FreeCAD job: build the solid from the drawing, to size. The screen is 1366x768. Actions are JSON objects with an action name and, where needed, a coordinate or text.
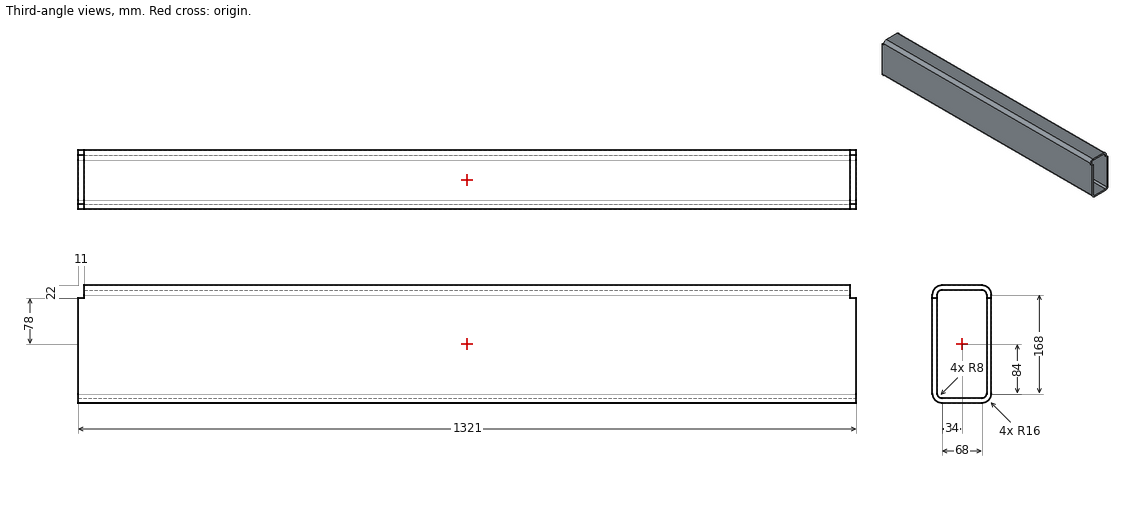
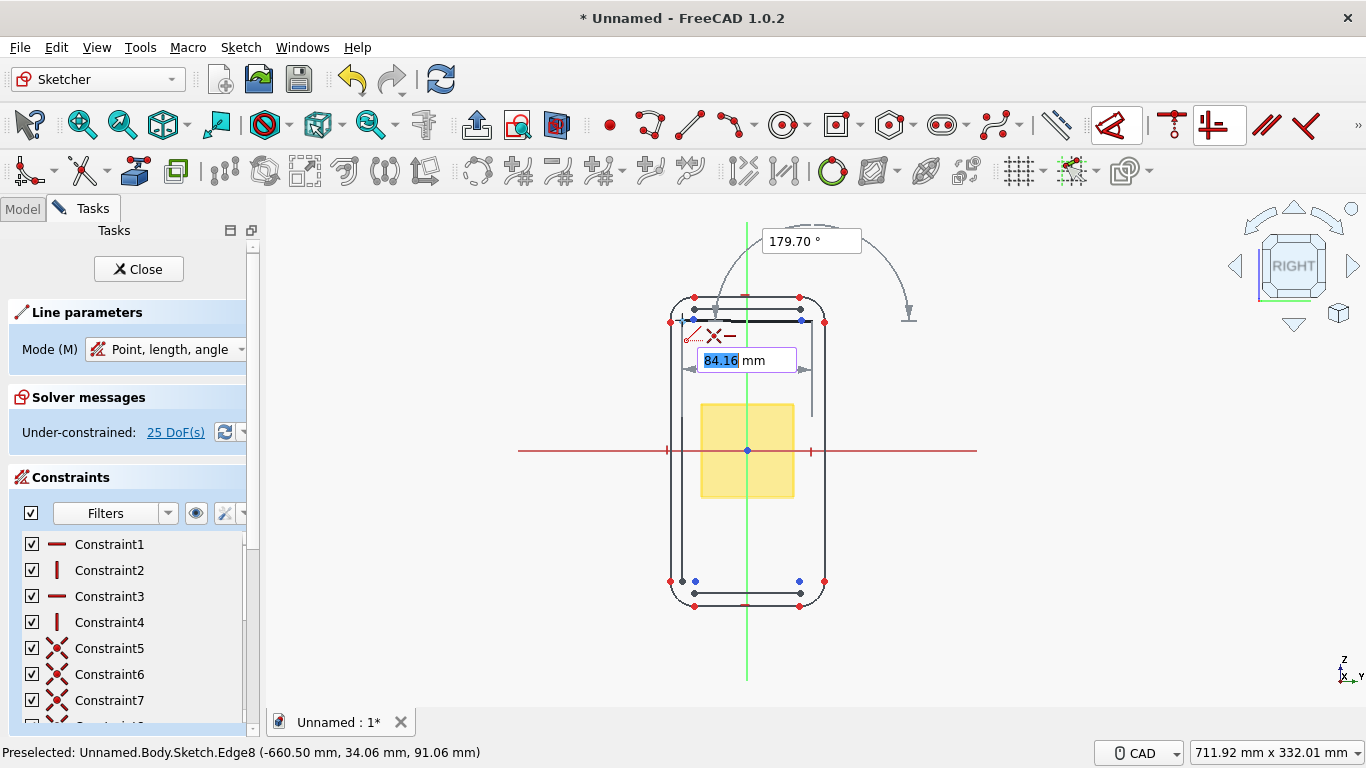
{"action": "scroll", "coordinate": [812, 581], "scroll_direction": "up", "scroll_amount": 2}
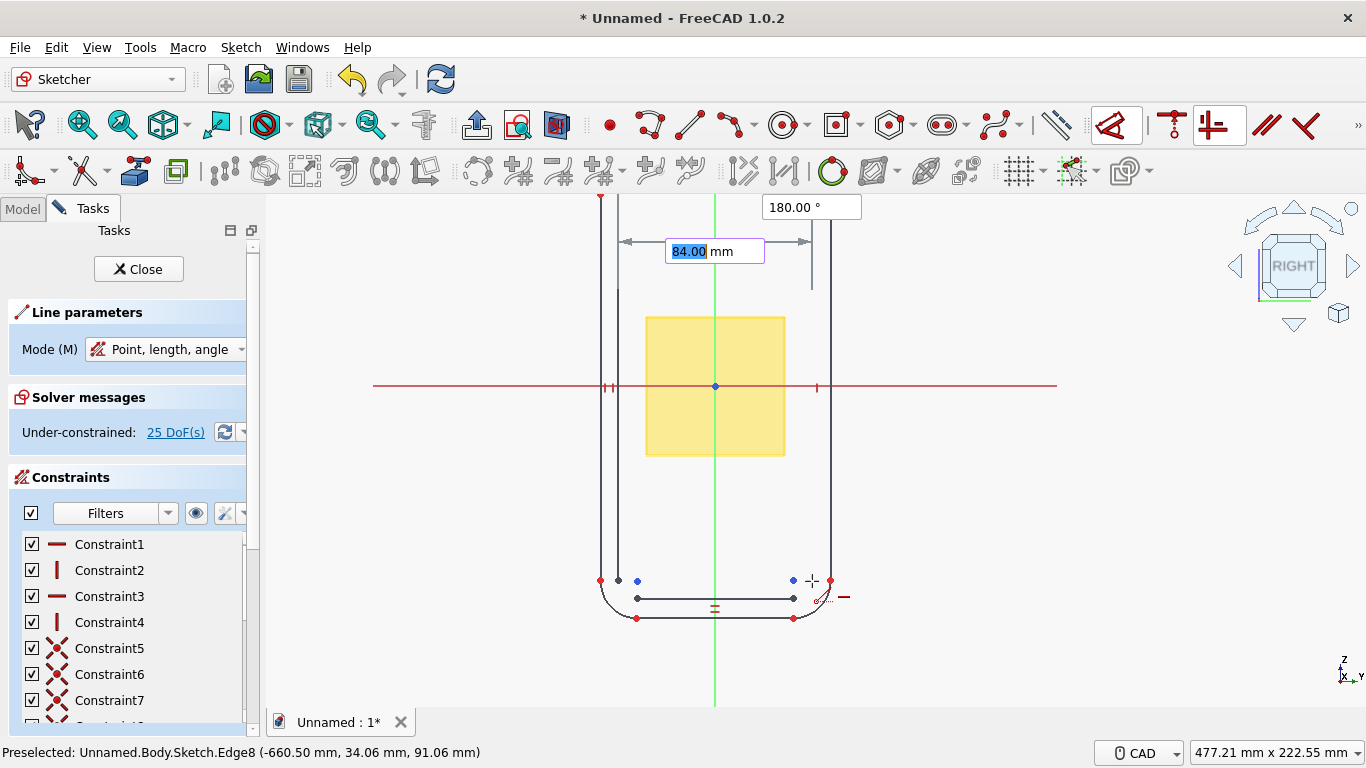
{"action": "left_click", "coordinate": [812, 580]}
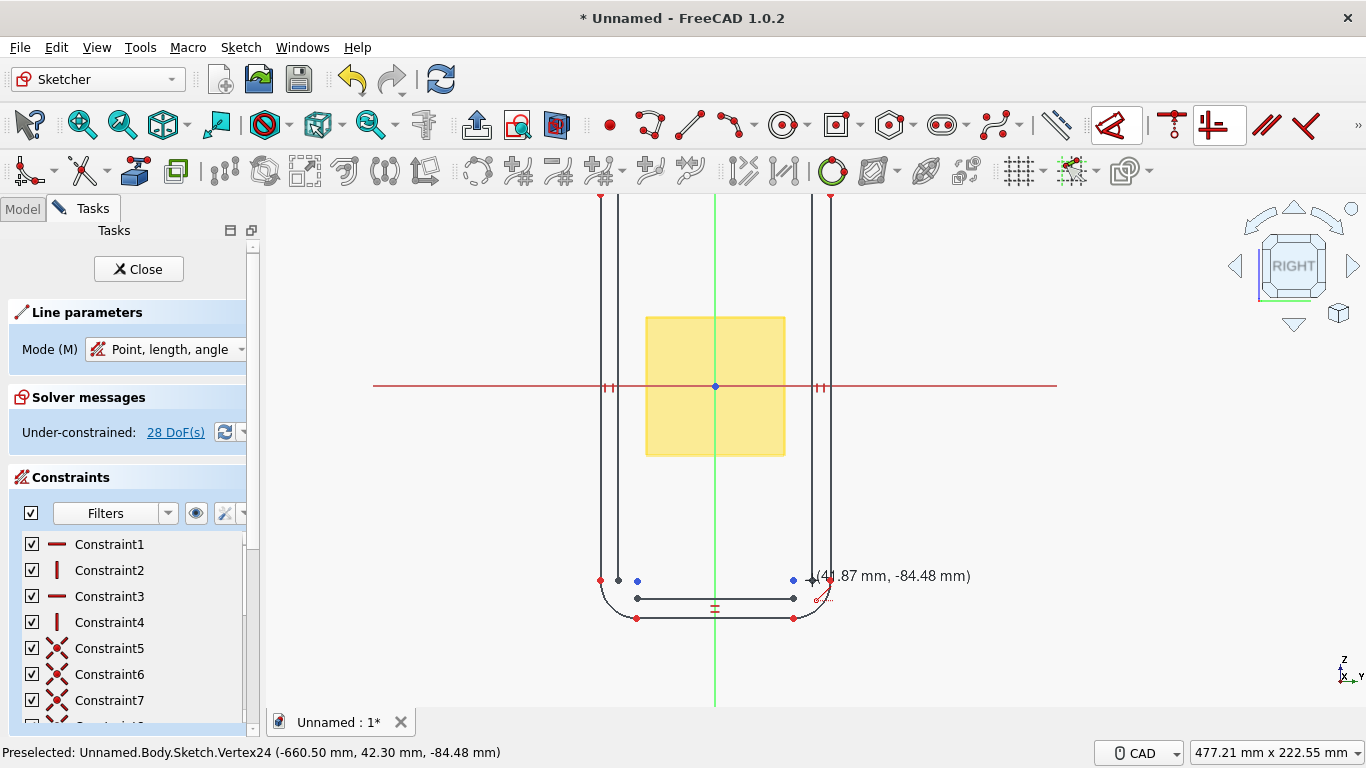
{"action": "left_click", "coordinate": [730, 126]}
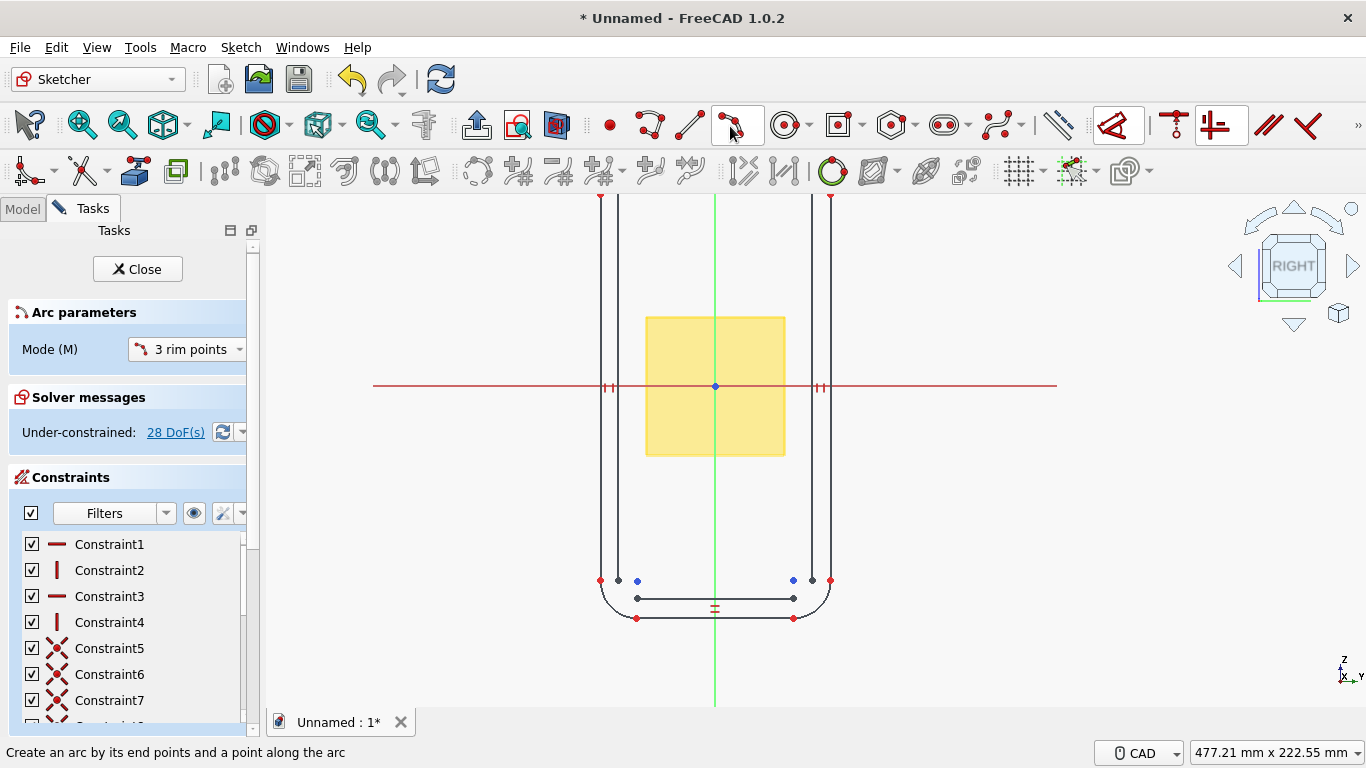
{"action": "left_click", "coordinate": [637, 599]}
{"action": "left_click", "coordinate": [618, 581]}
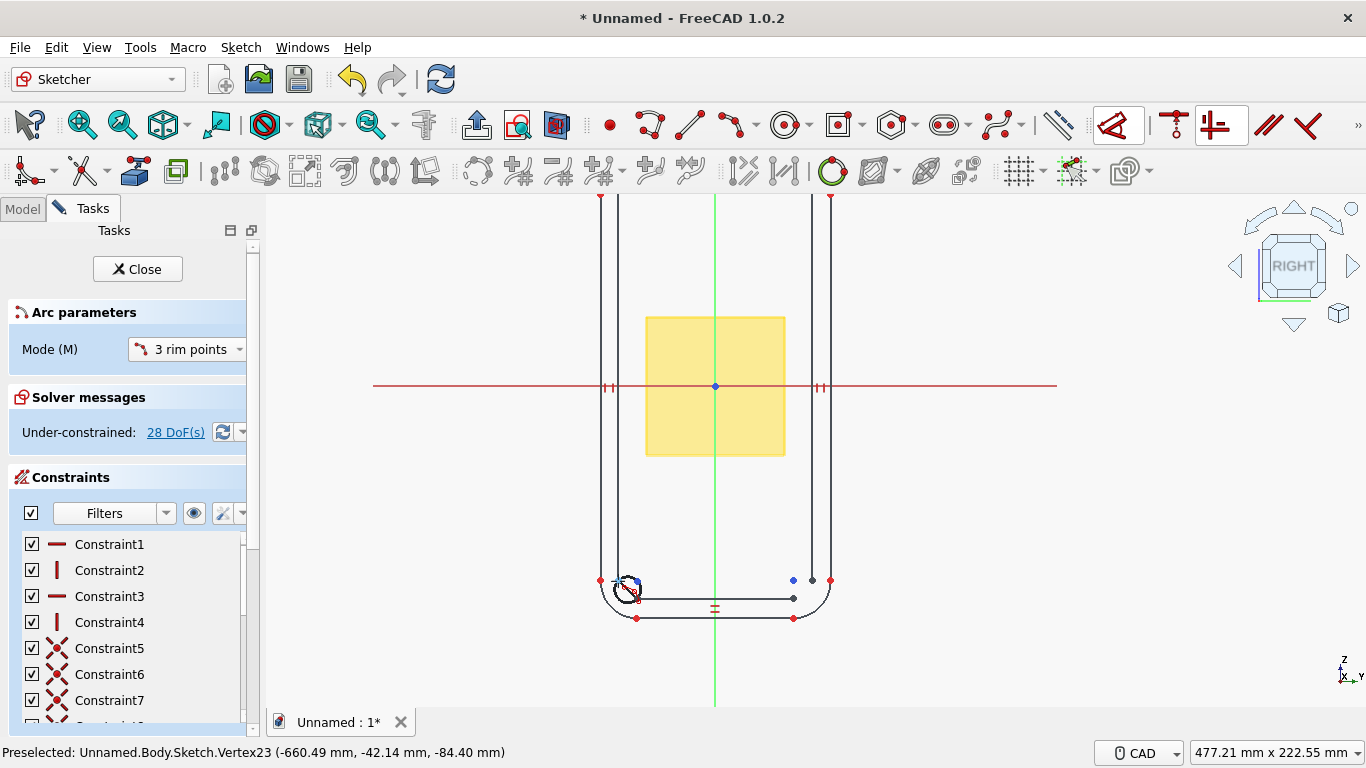
{"action": "scroll", "coordinate": [624, 593], "scroll_direction": "up", "scroll_amount": 6}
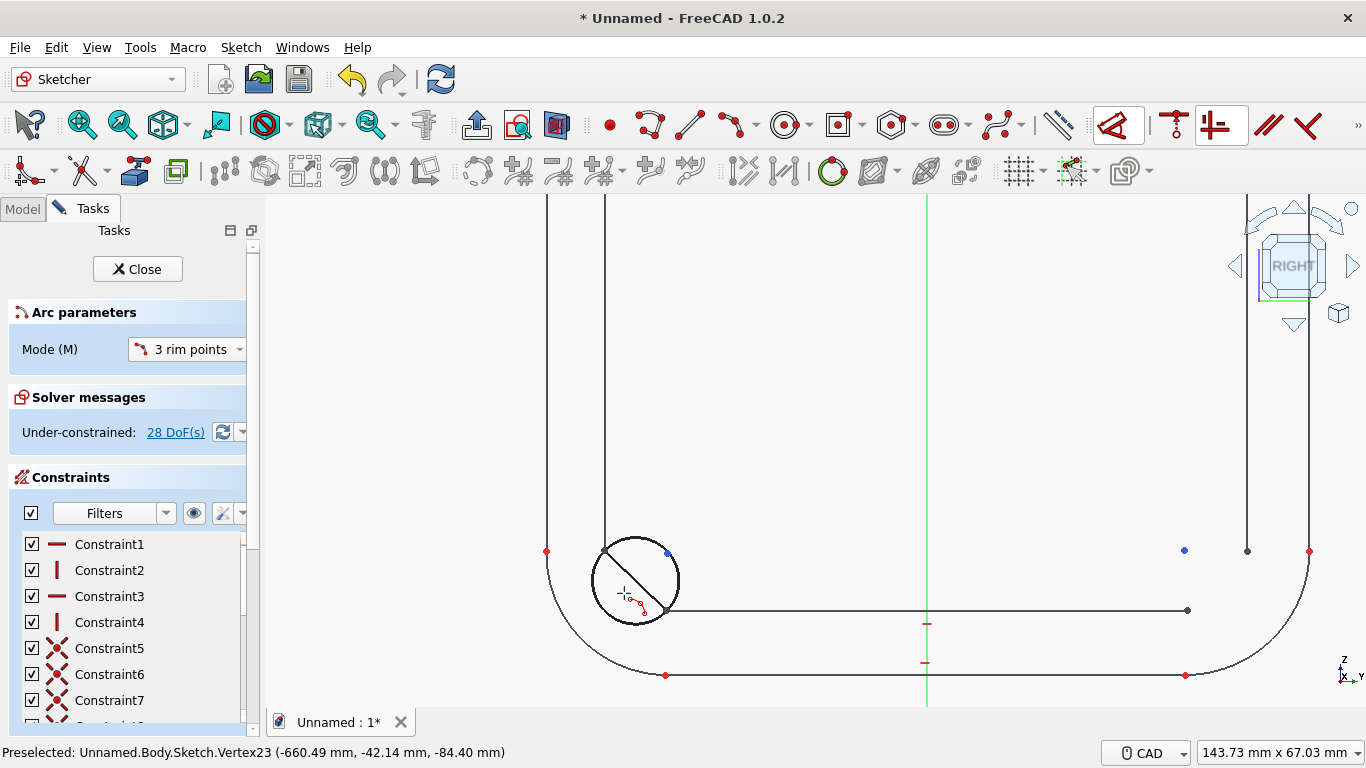
{"action": "left_click", "coordinate": [624, 591]}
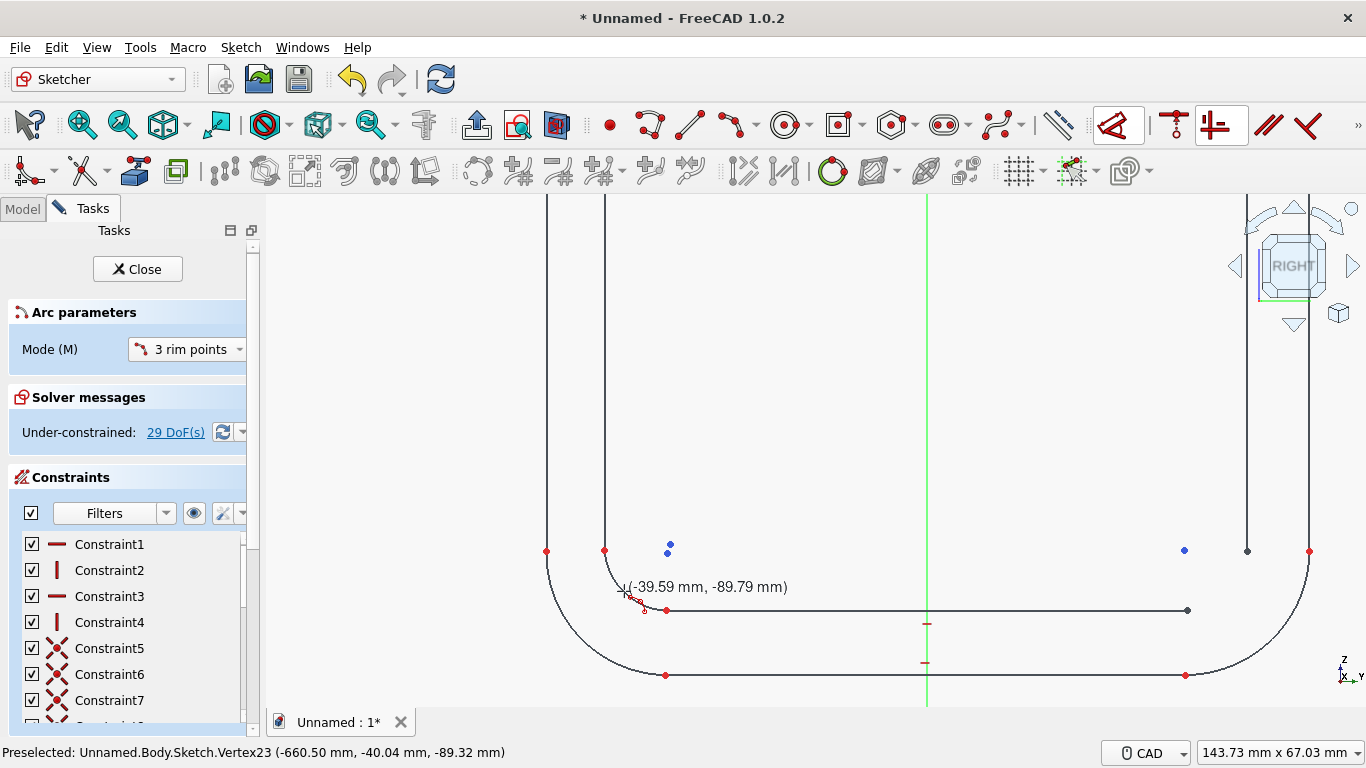
{"action": "scroll", "coordinate": [702, 589], "scroll_direction": "down", "scroll_amount": 8}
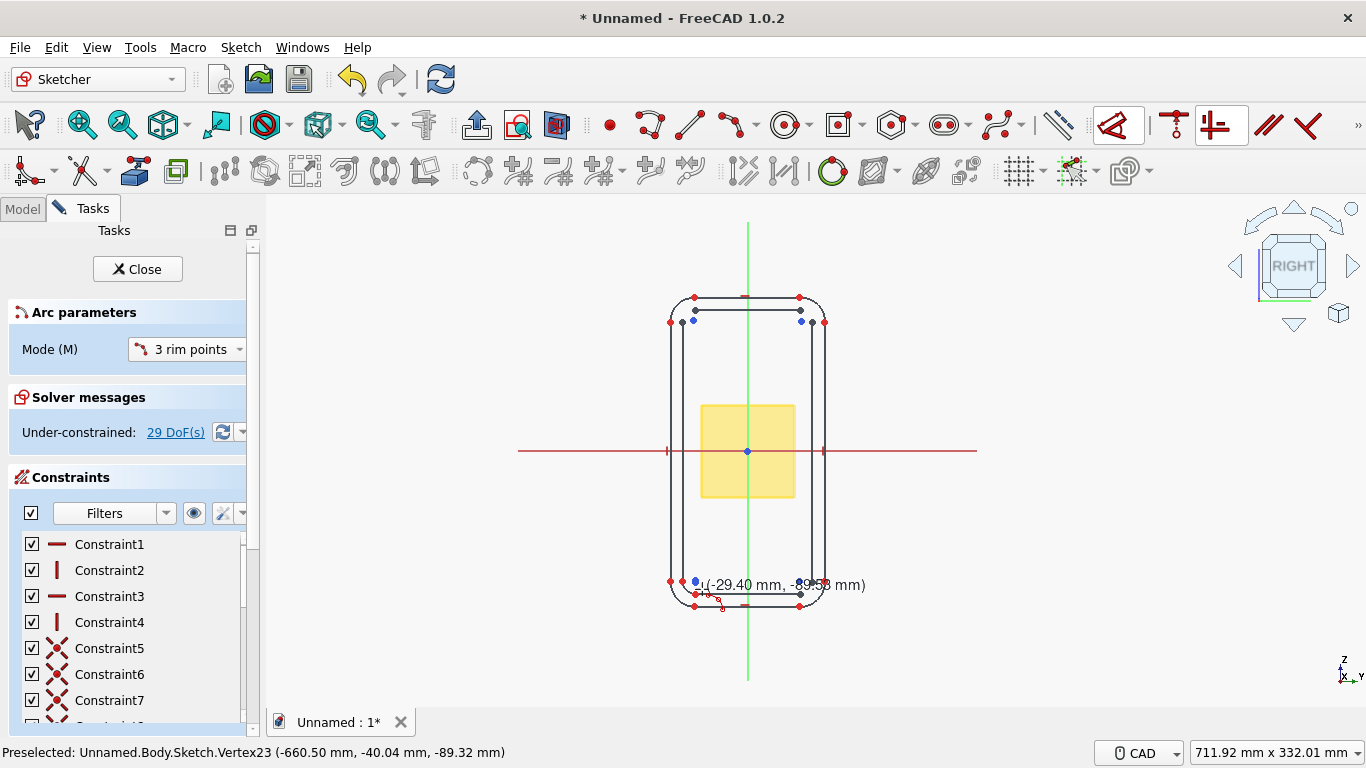
{"action": "scroll", "coordinate": [683, 322], "scroll_direction": "up", "scroll_amount": 2}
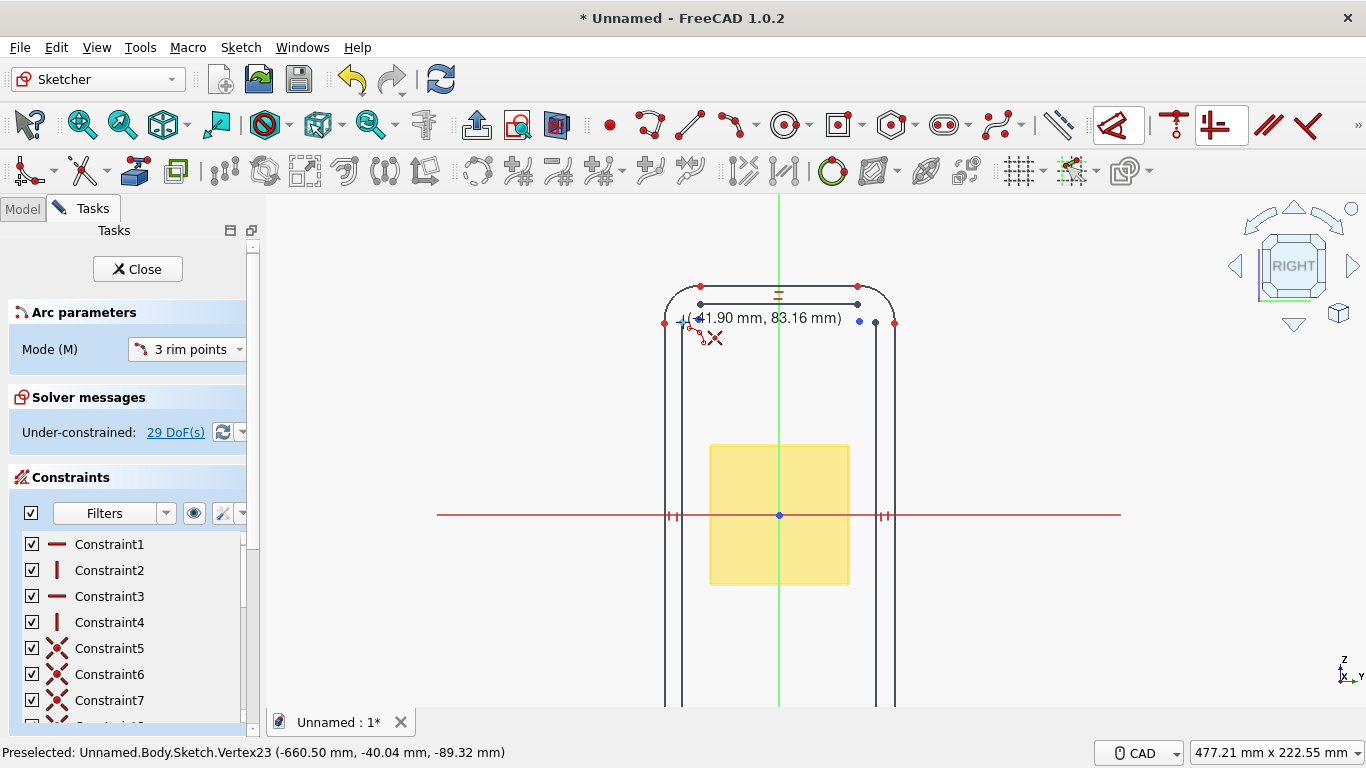
{"action": "left_click", "coordinate": [682, 322]}
{"action": "left_click", "coordinate": [701, 304]}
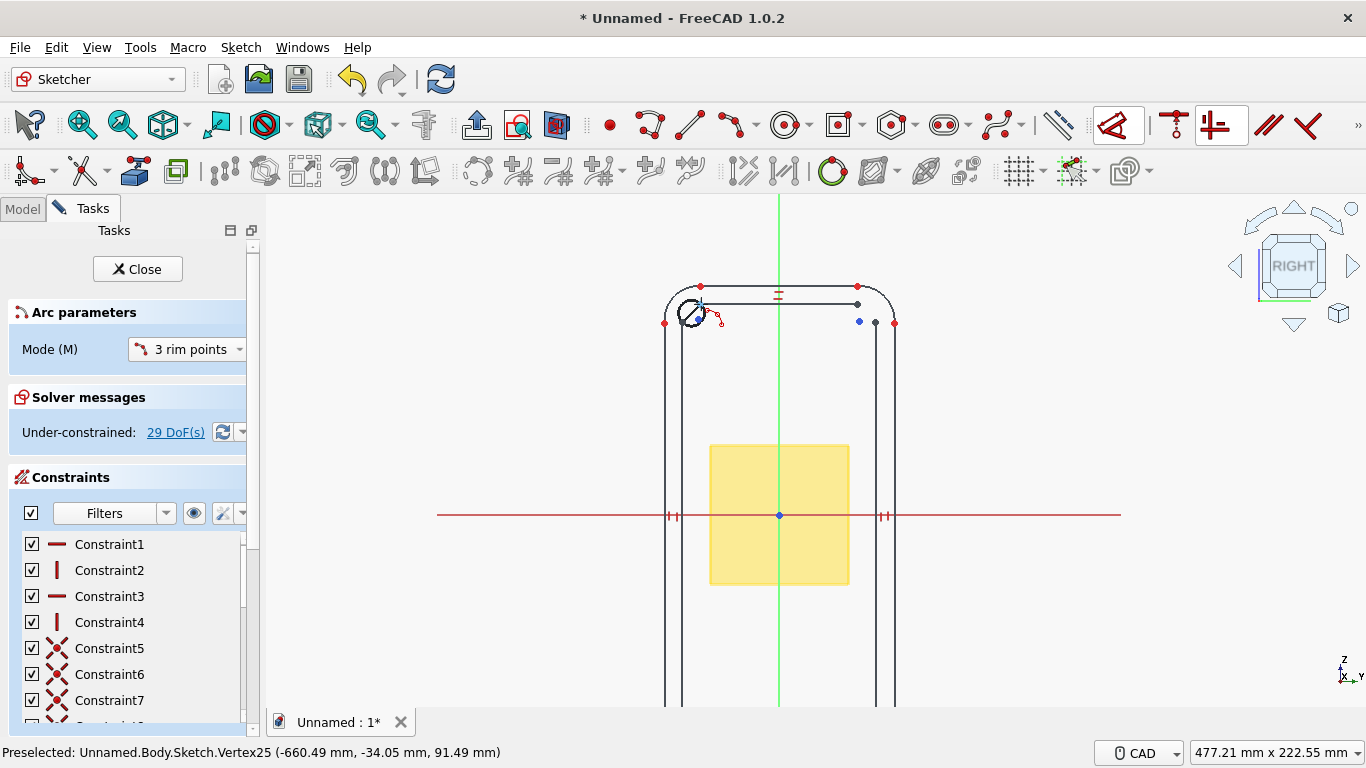
{"action": "scroll", "coordinate": [688, 308], "scroll_direction": "up", "scroll_amount": 6}